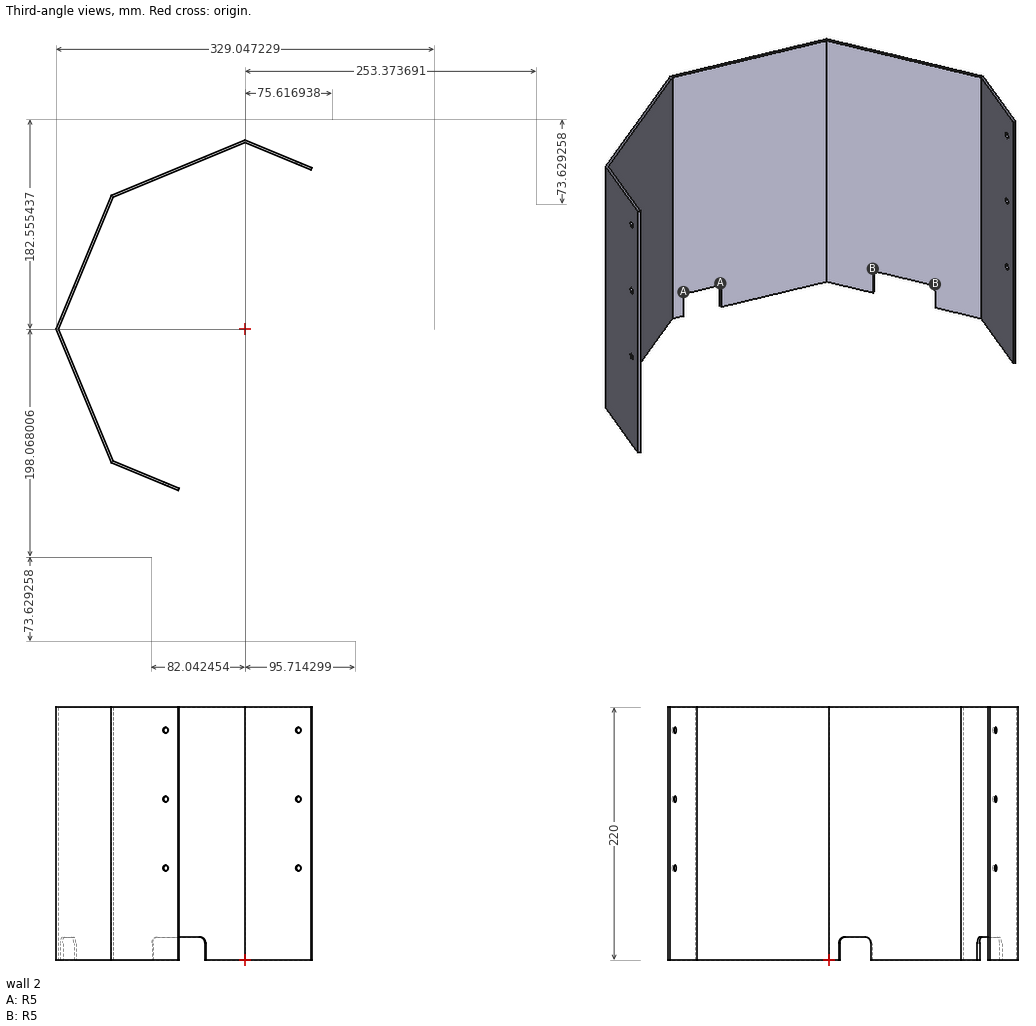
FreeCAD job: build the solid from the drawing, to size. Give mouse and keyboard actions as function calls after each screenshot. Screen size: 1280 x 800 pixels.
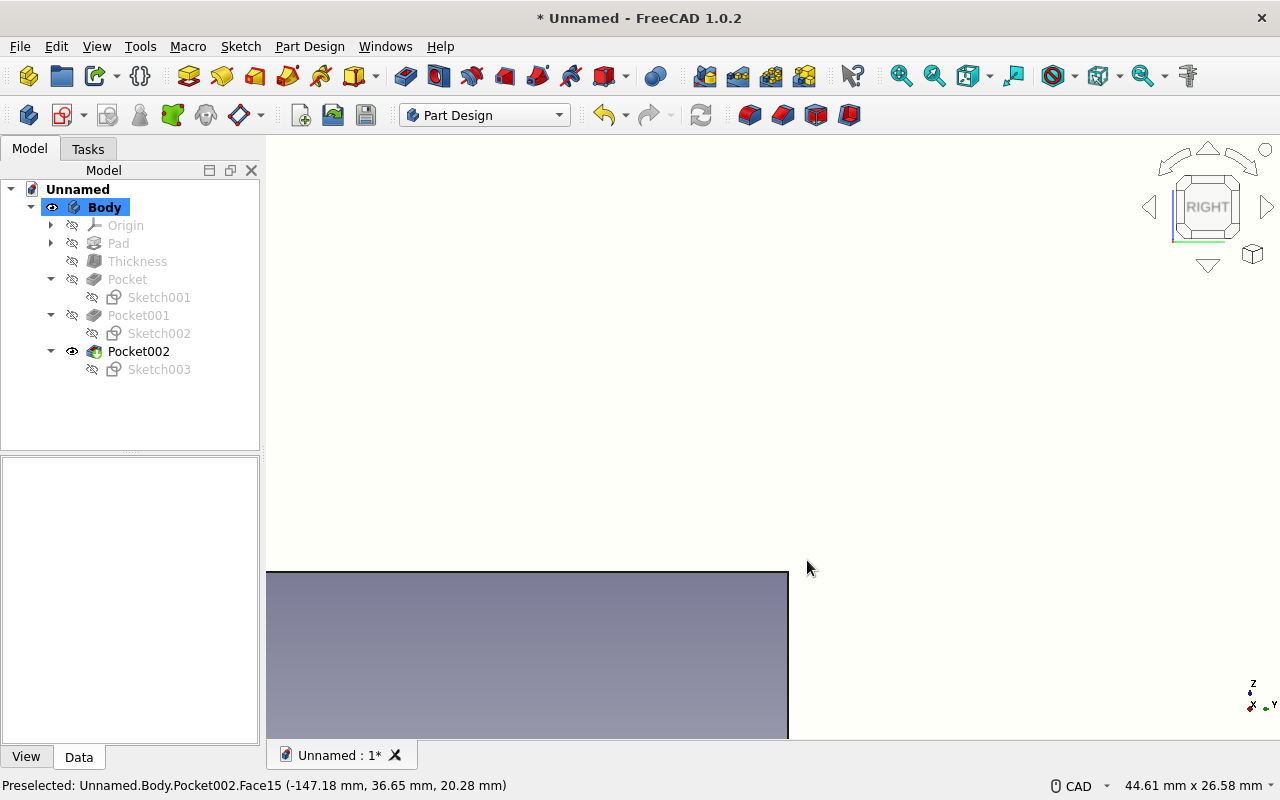
click(902, 76)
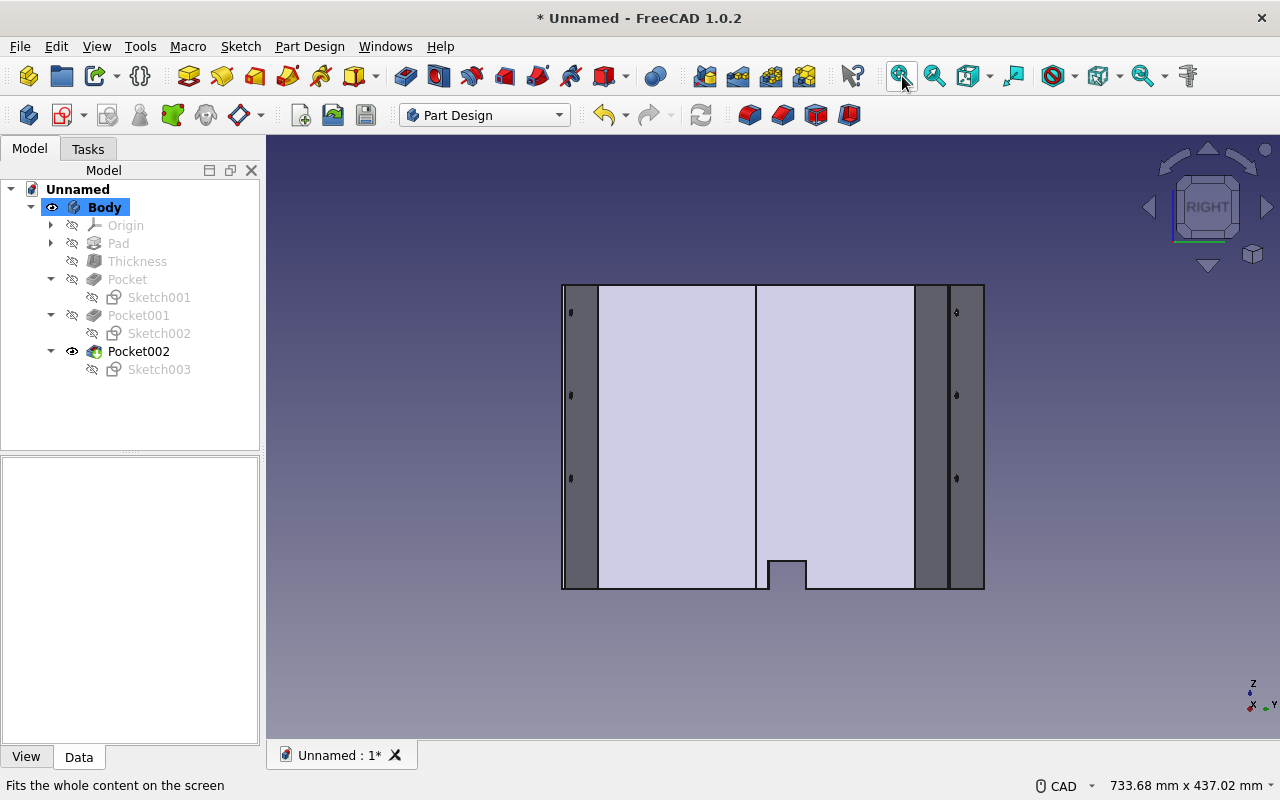
key(5)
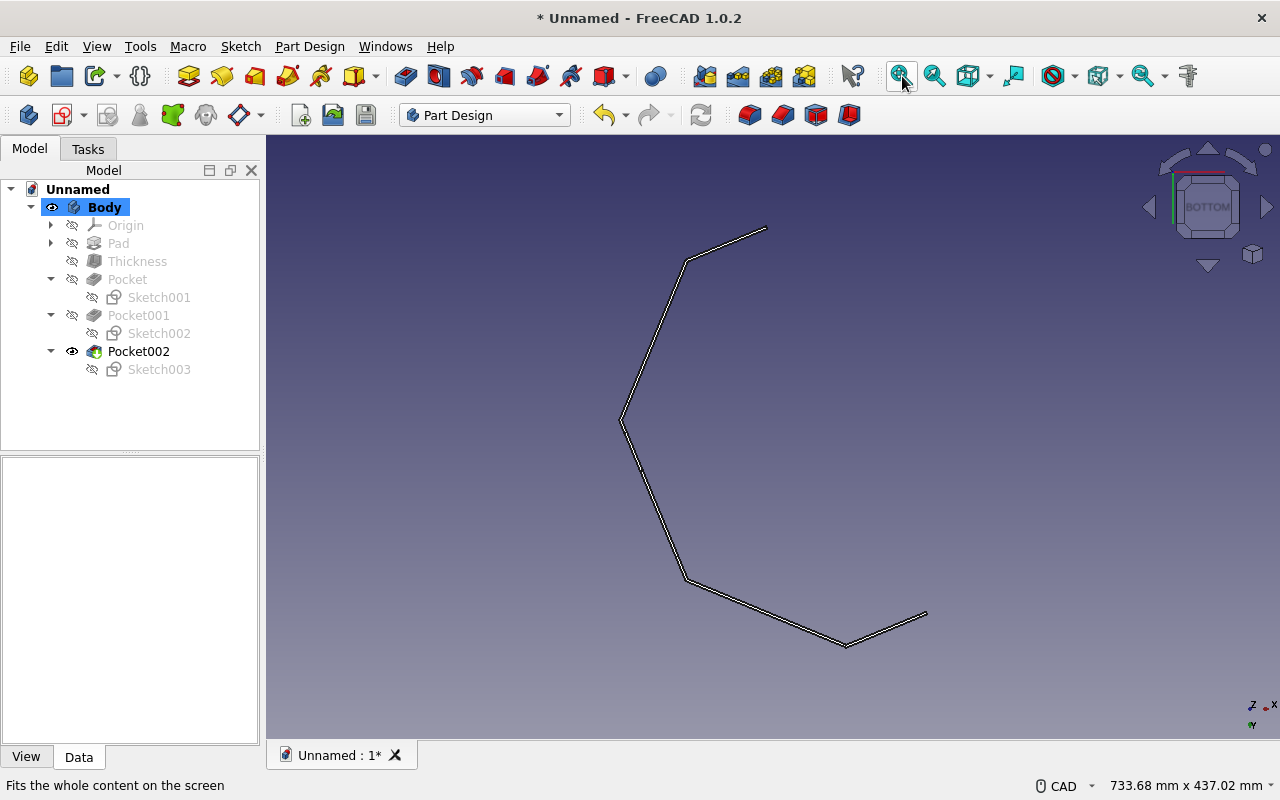
scroll(642, 470, up, 14)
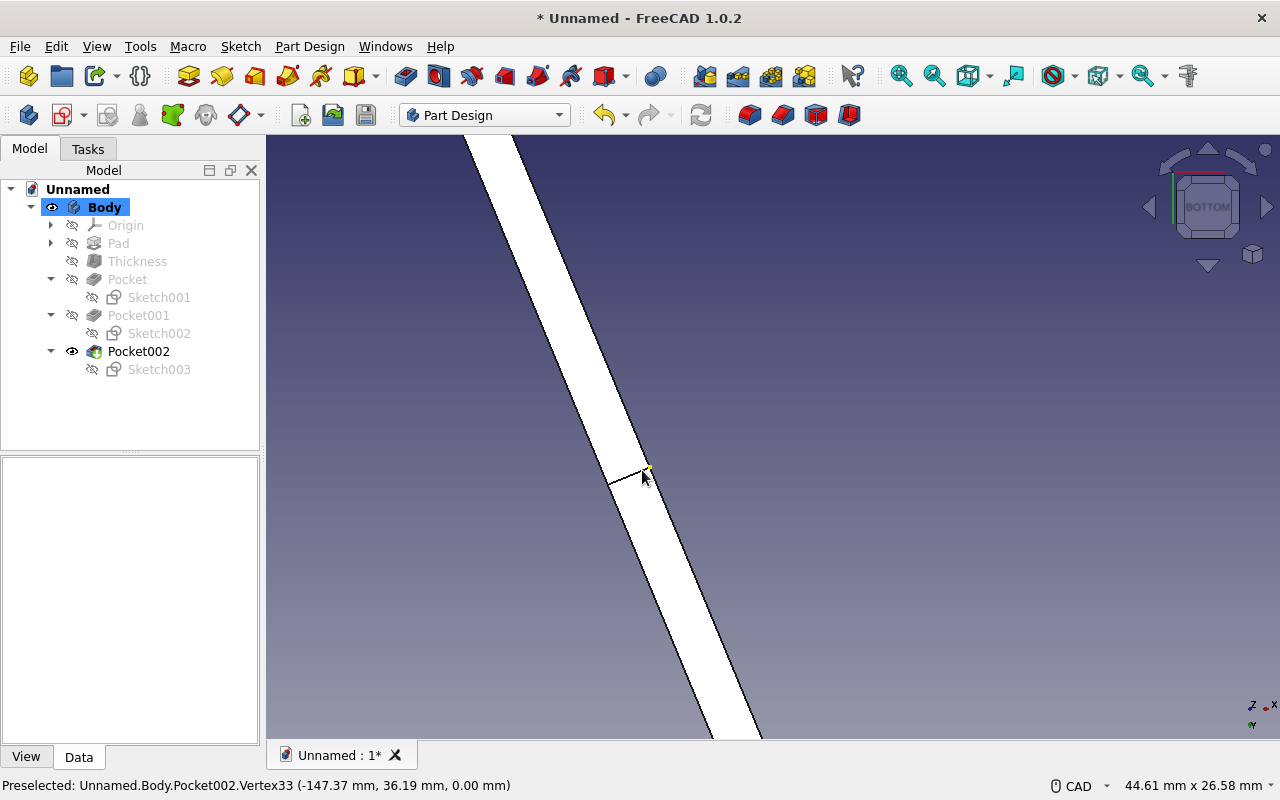
click(902, 76)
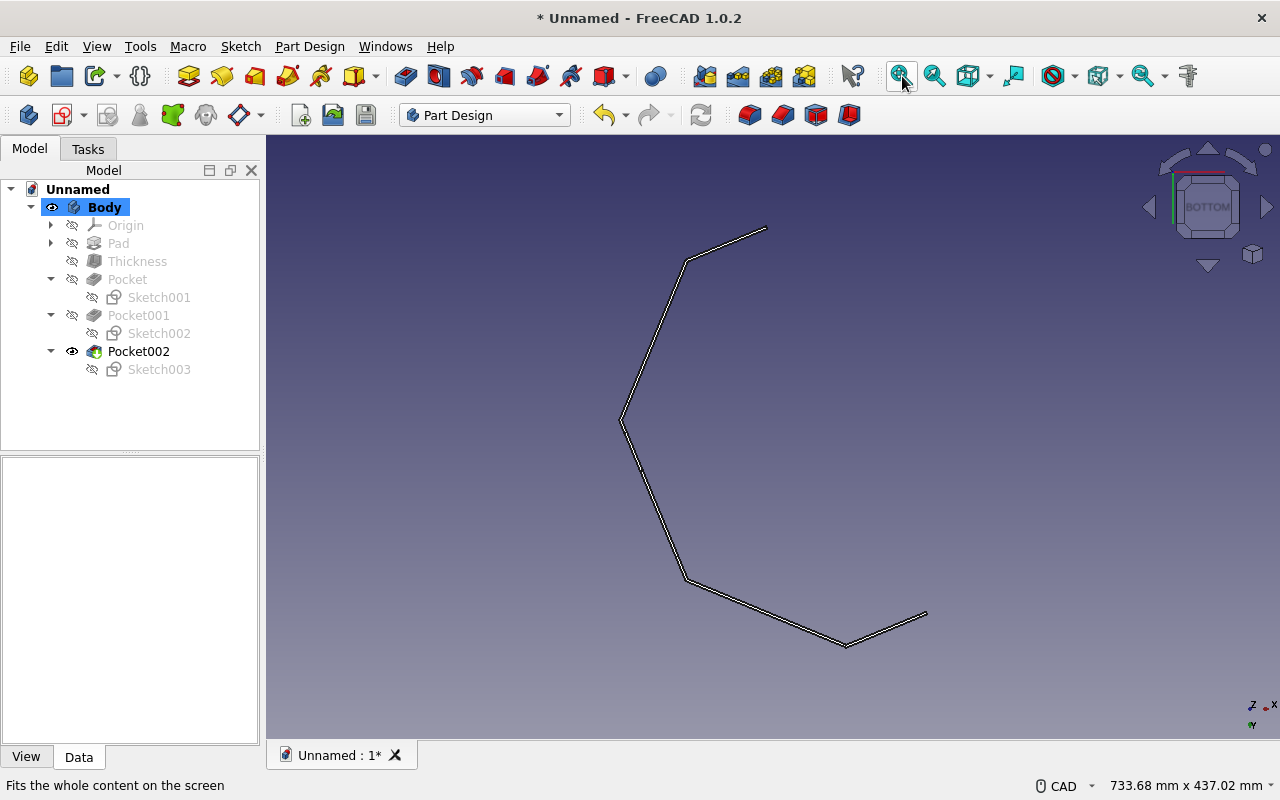
key(4)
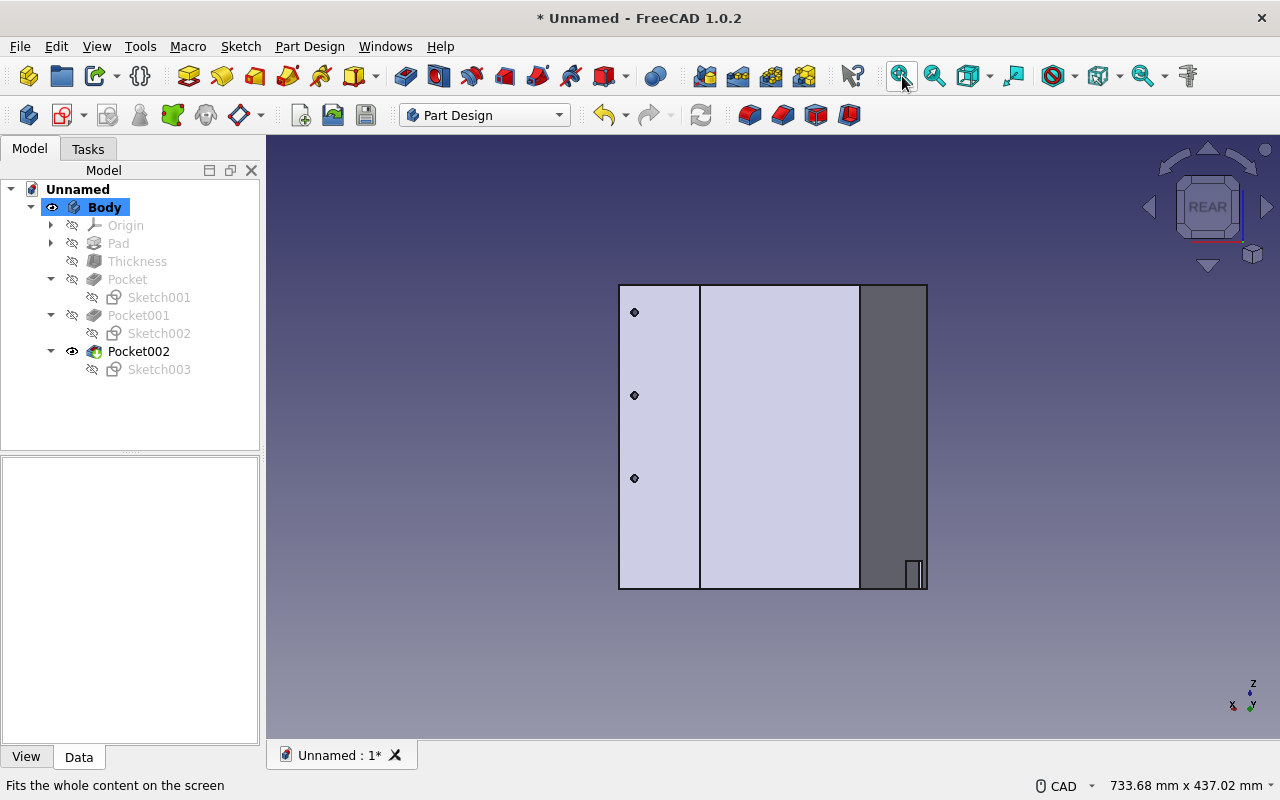
scroll(904, 560, up, 14)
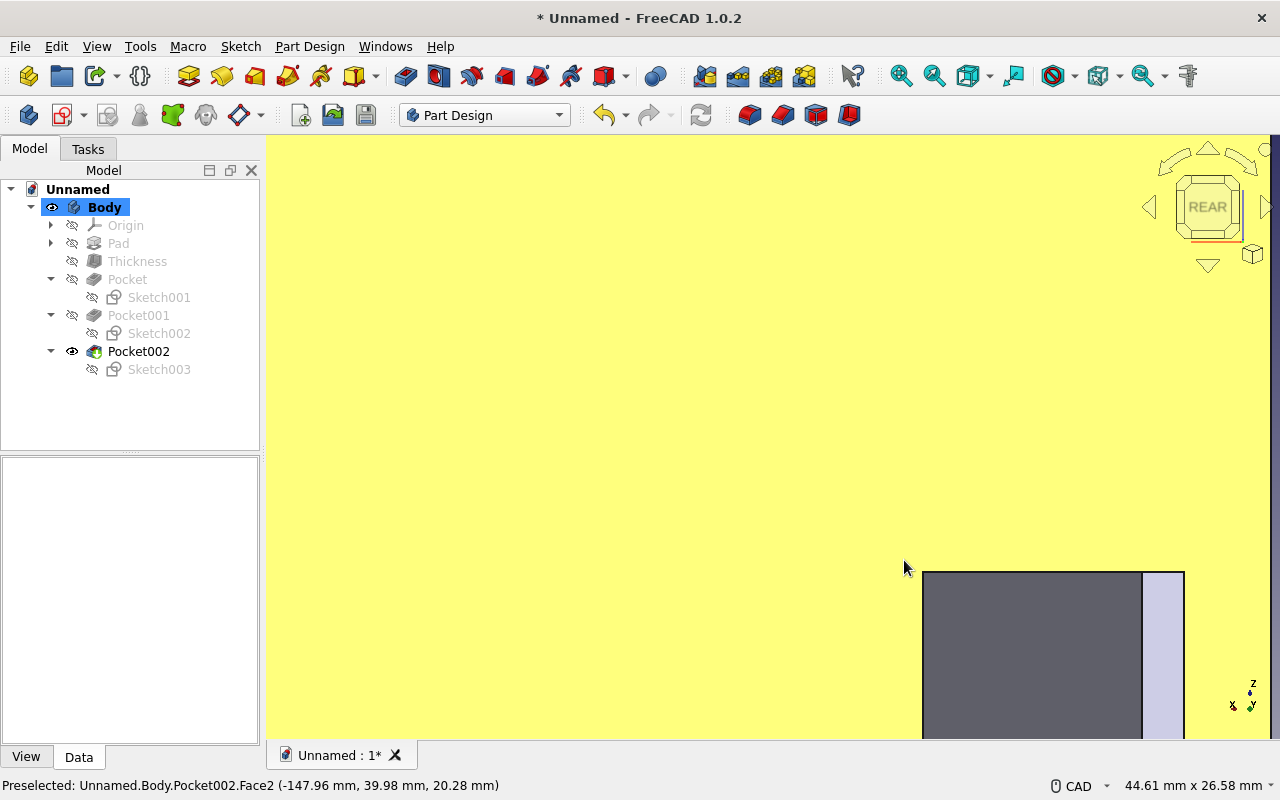
click(902, 76)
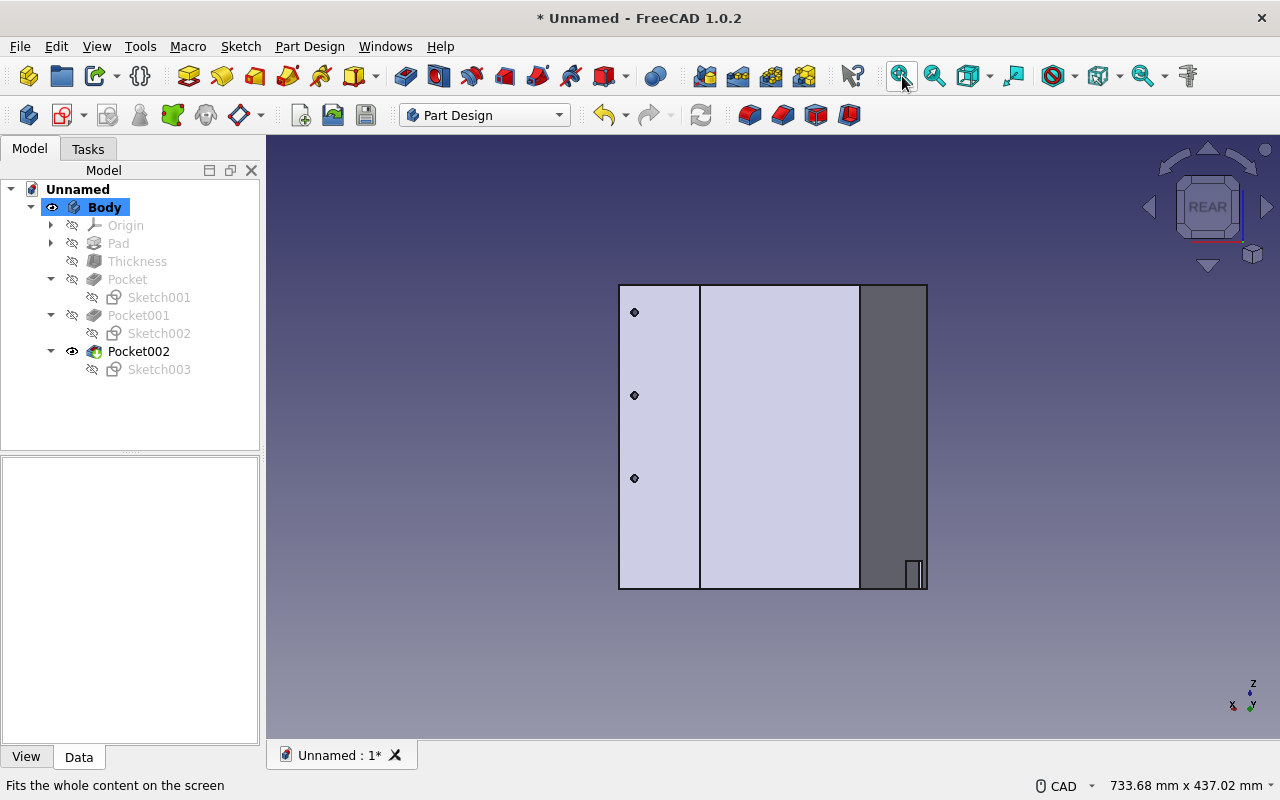
key(6)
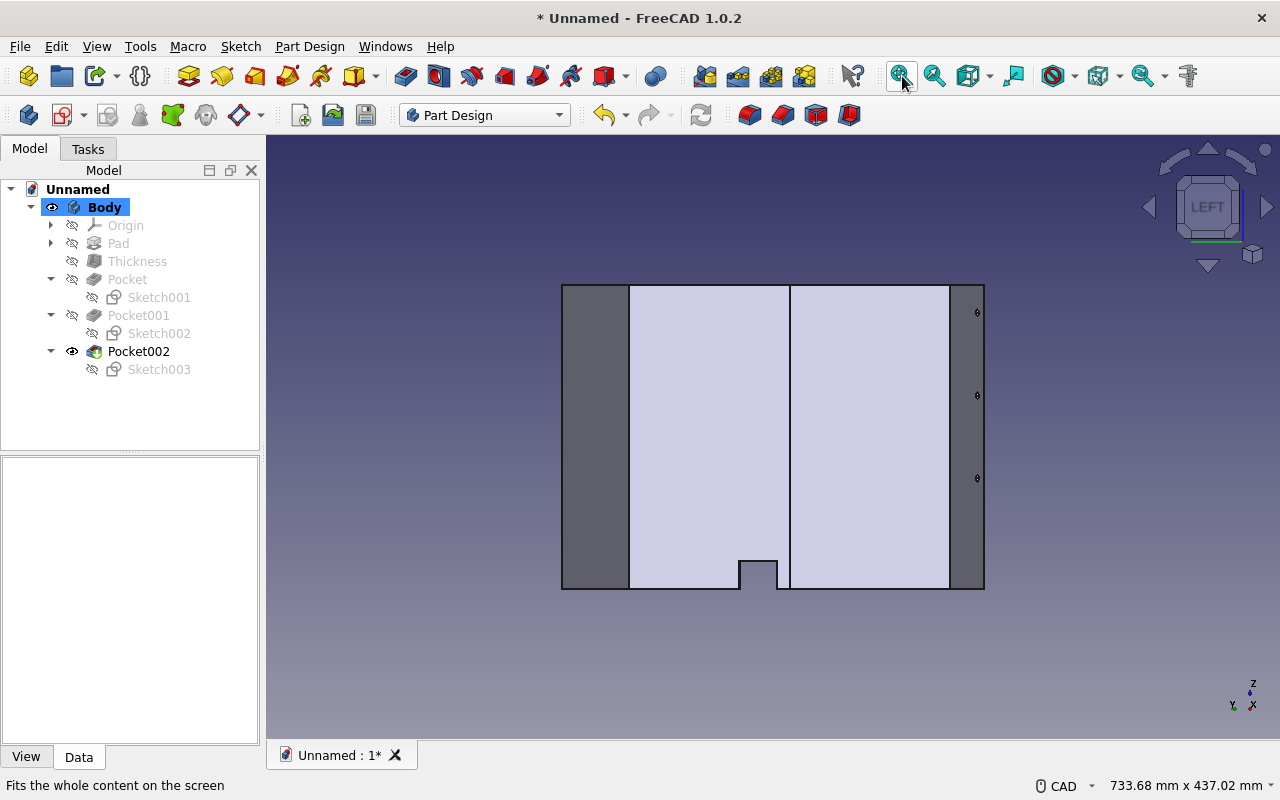
scroll(739, 560, up, 14)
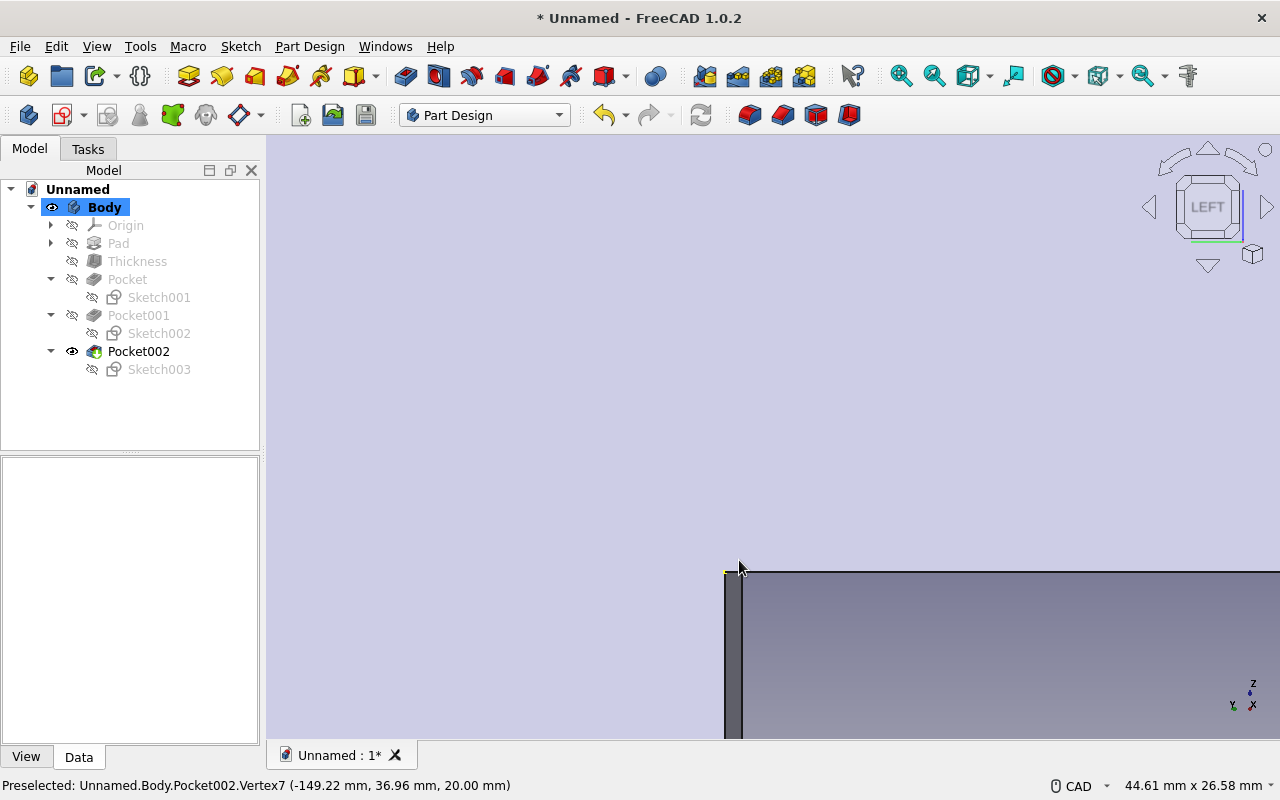
click(902, 76)